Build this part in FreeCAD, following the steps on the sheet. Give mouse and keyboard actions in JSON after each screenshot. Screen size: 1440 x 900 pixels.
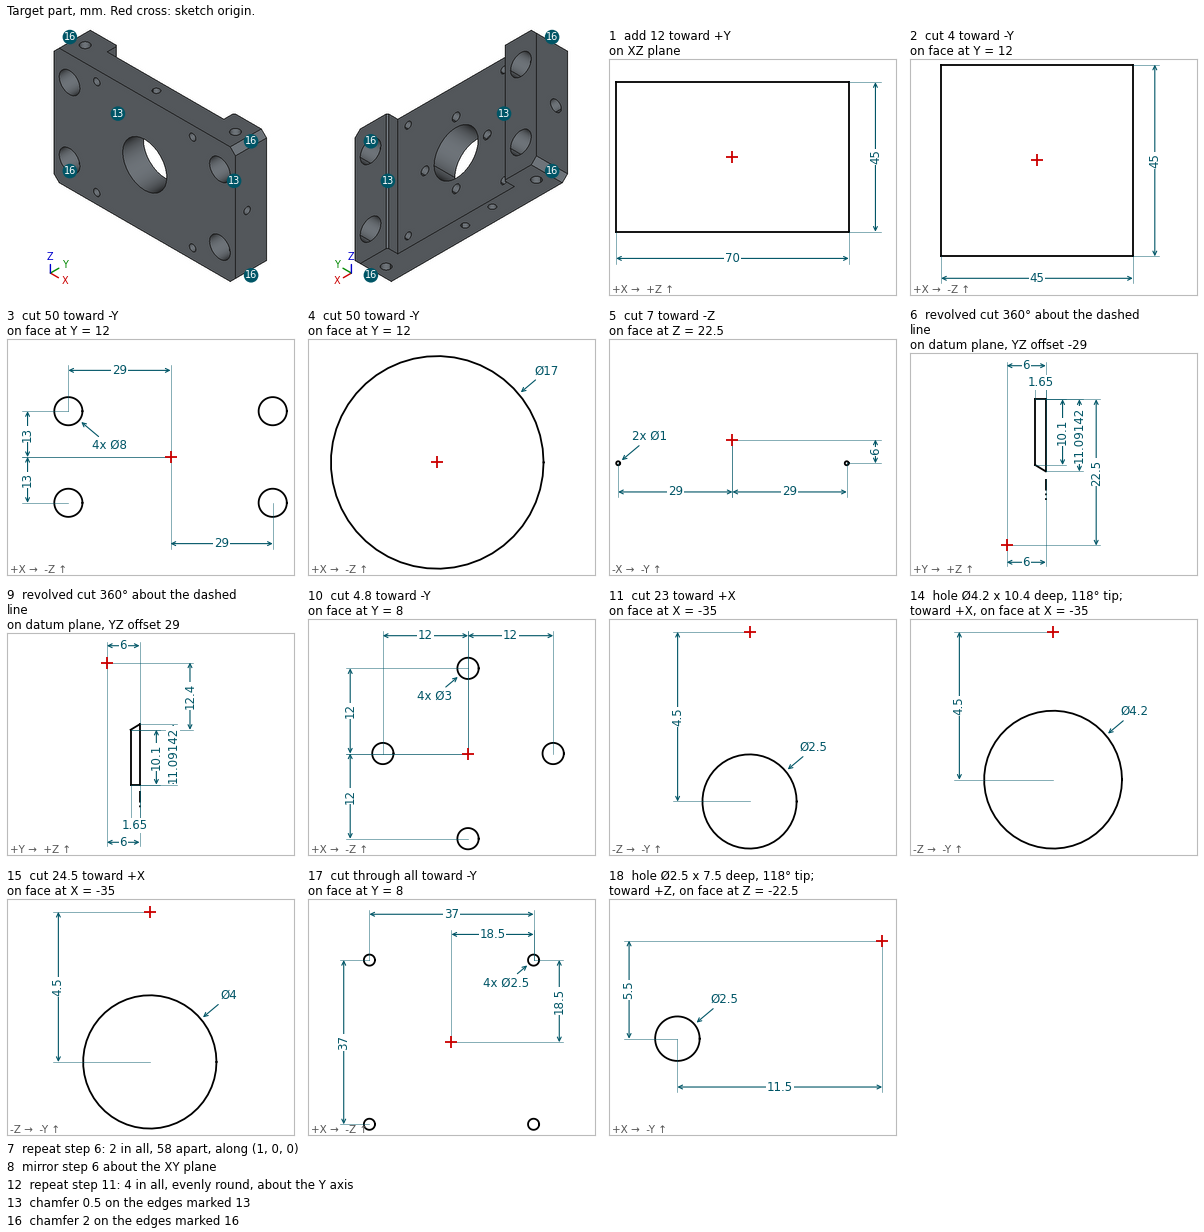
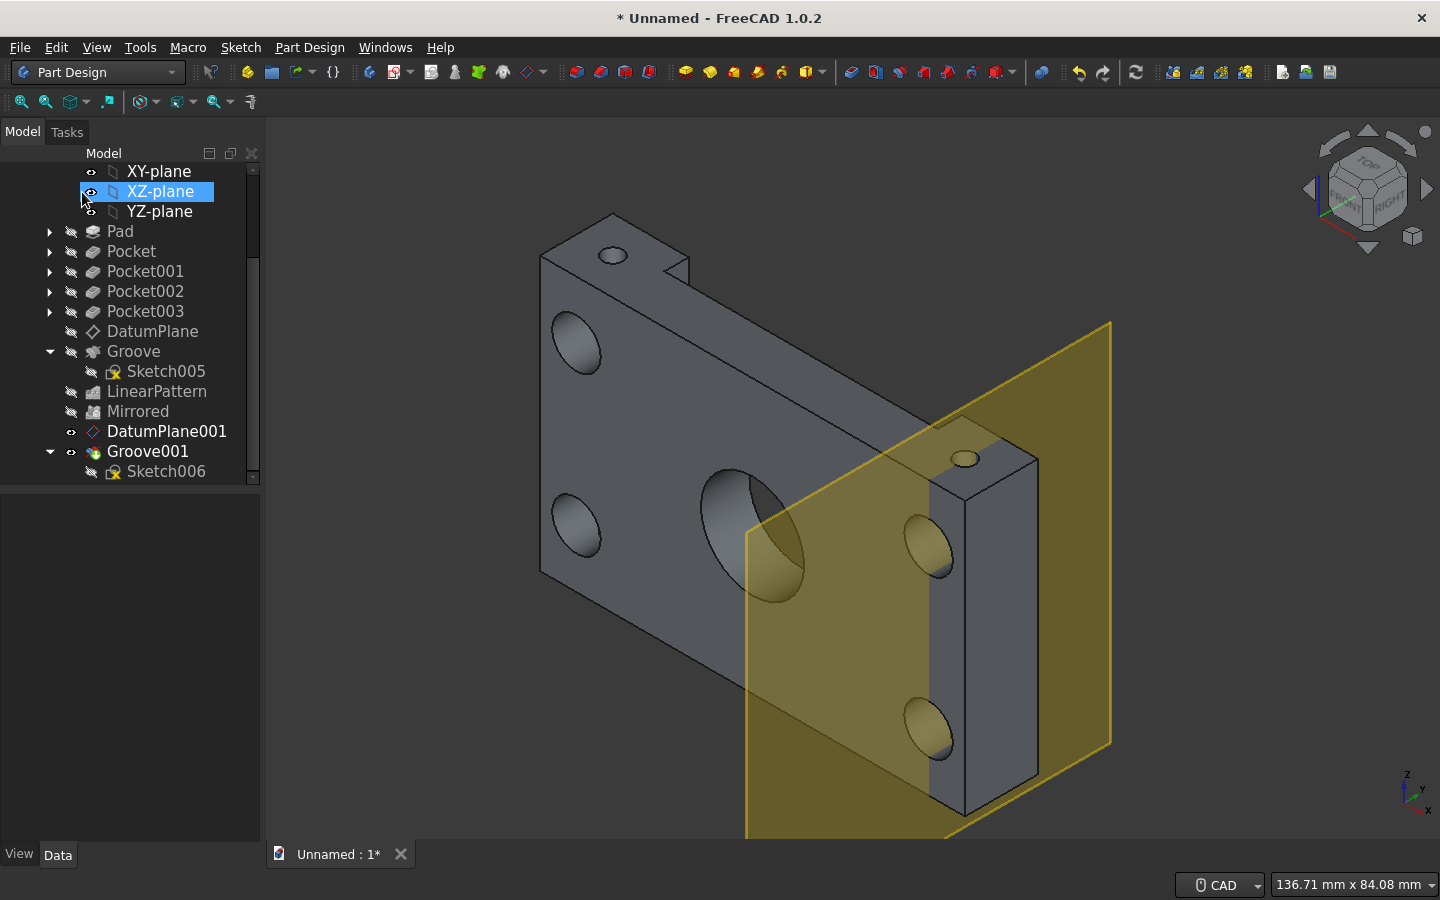
{"action": "left_click", "coordinate": [116, 432]}
{"action": "key", "text": "space"}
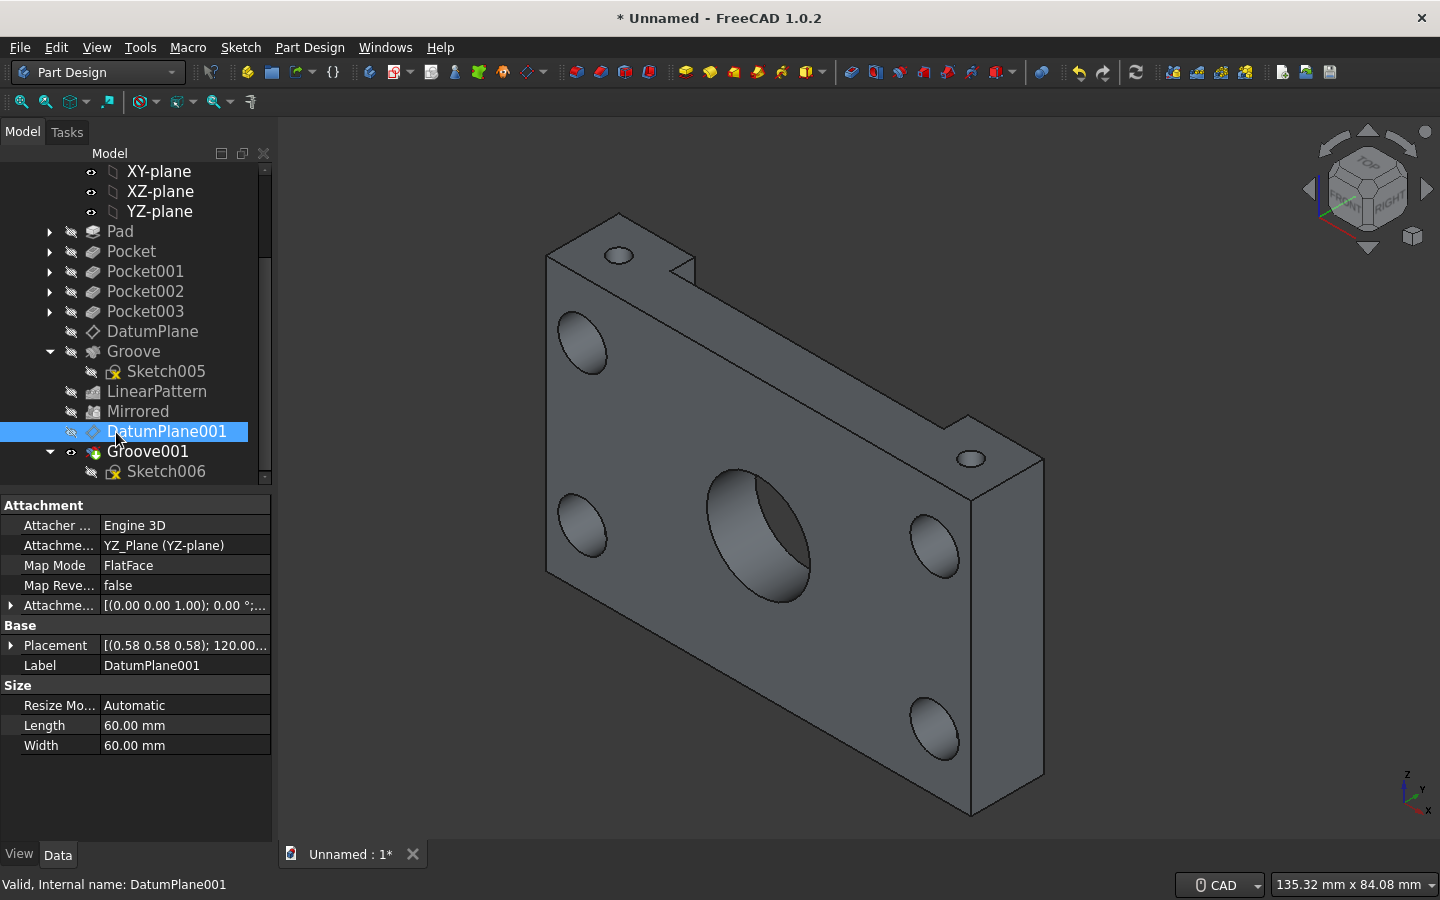
{"action": "key", "text": "4"}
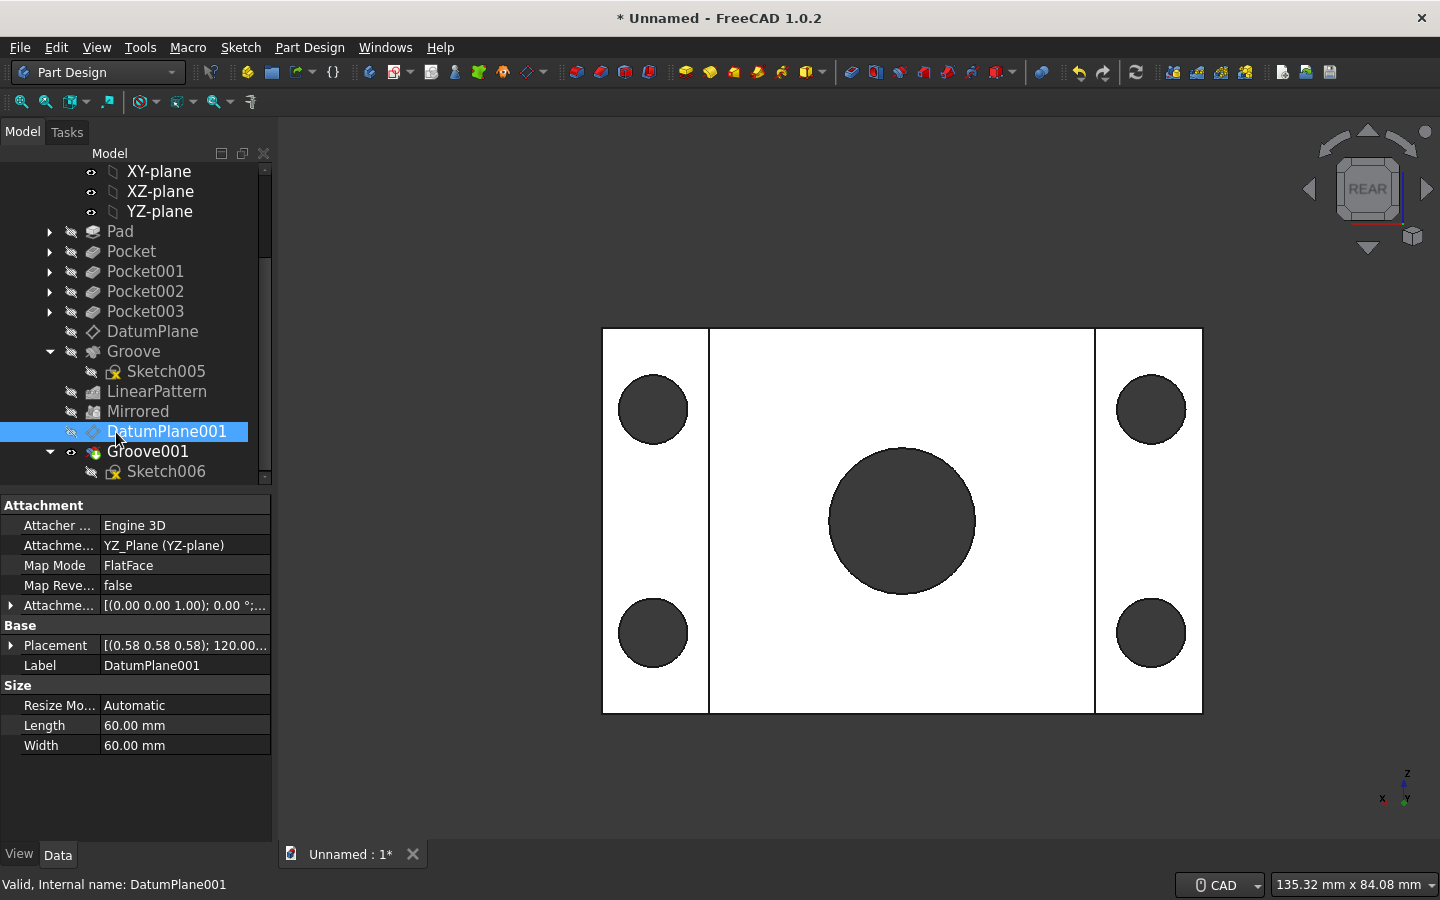
{"action": "left_click", "coordinate": [792, 410]}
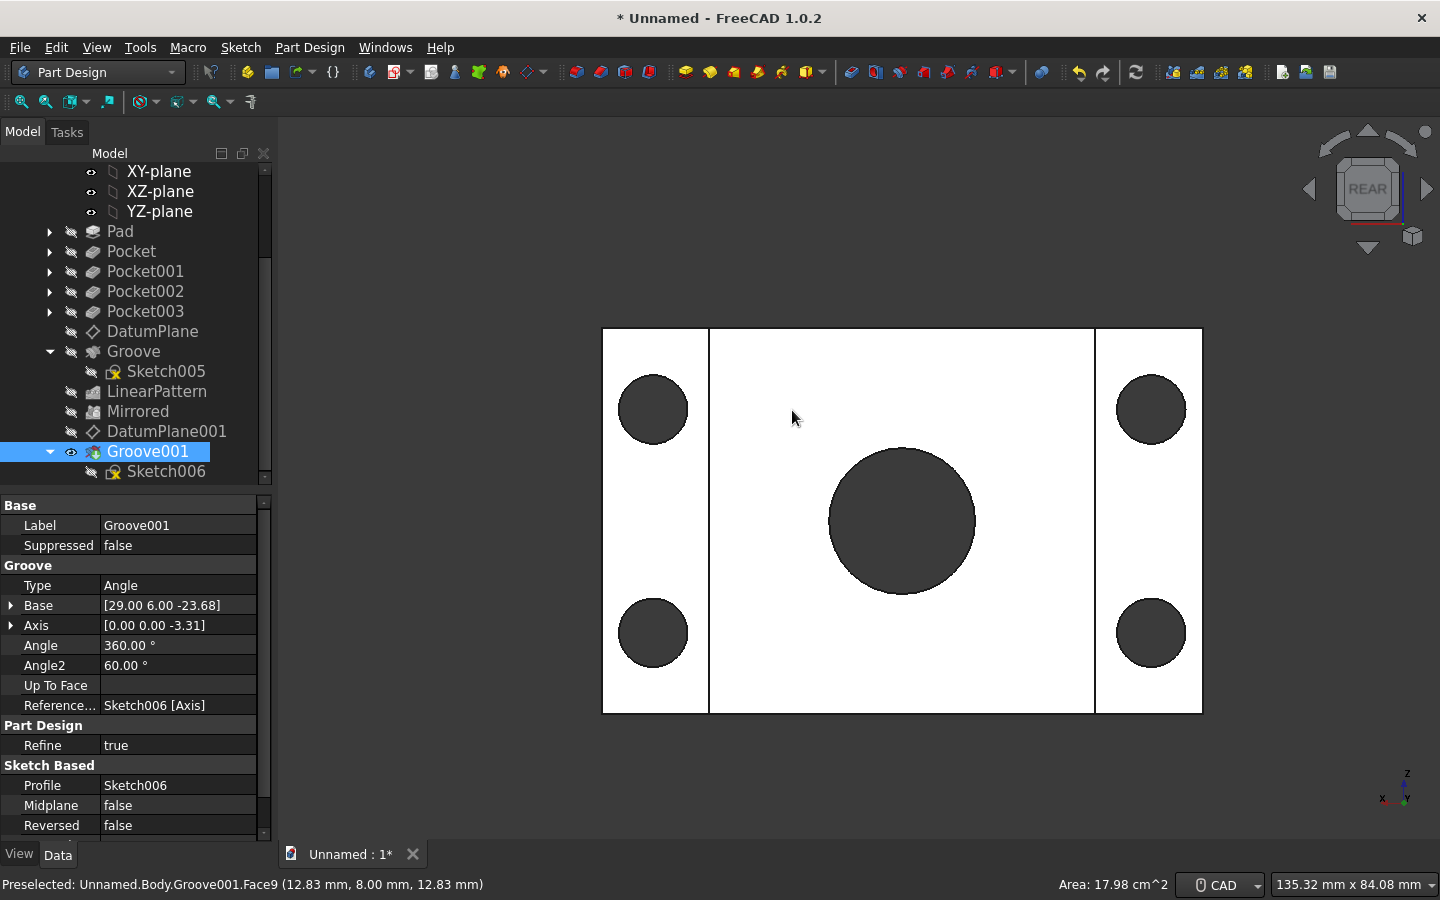
{"action": "left_click", "coordinate": [394, 72]}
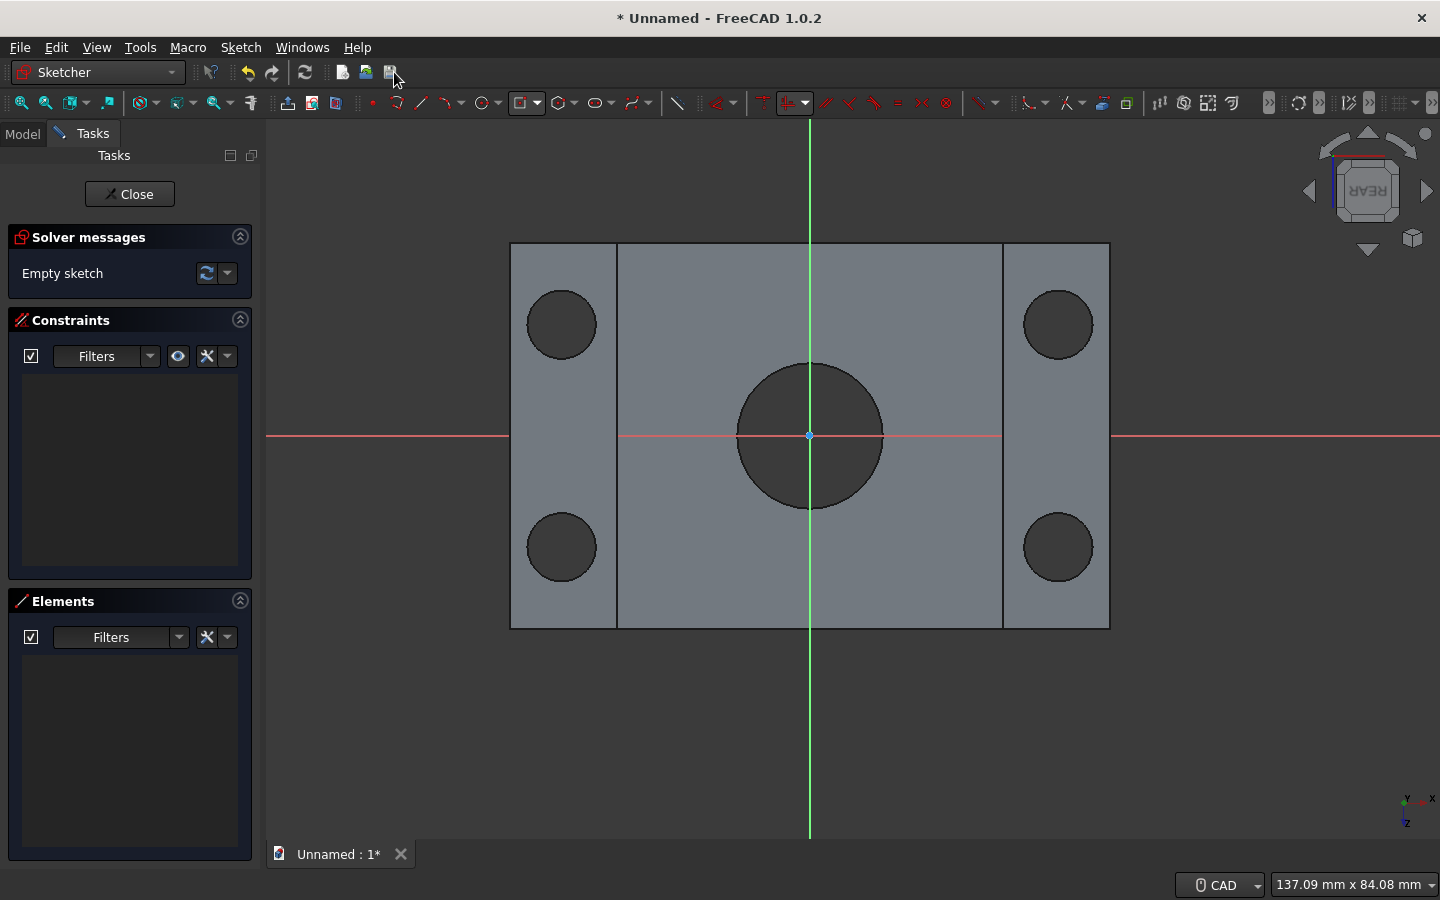
{"action": "left_click", "coordinate": [336, 104]}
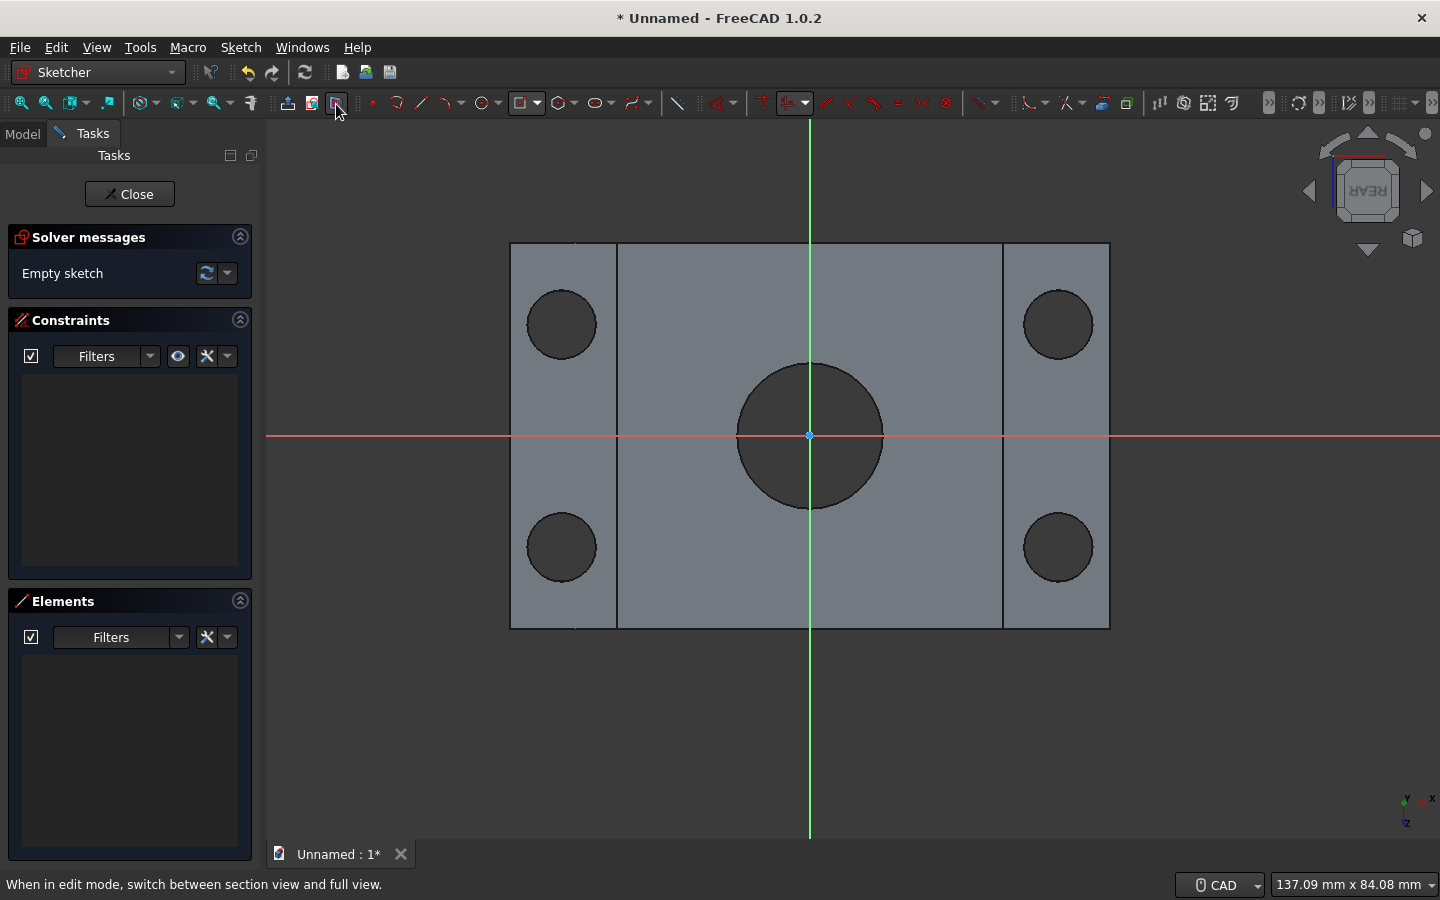
{"action": "scroll", "coordinate": [831, 401], "scroll_direction": "up", "scroll_amount": 4}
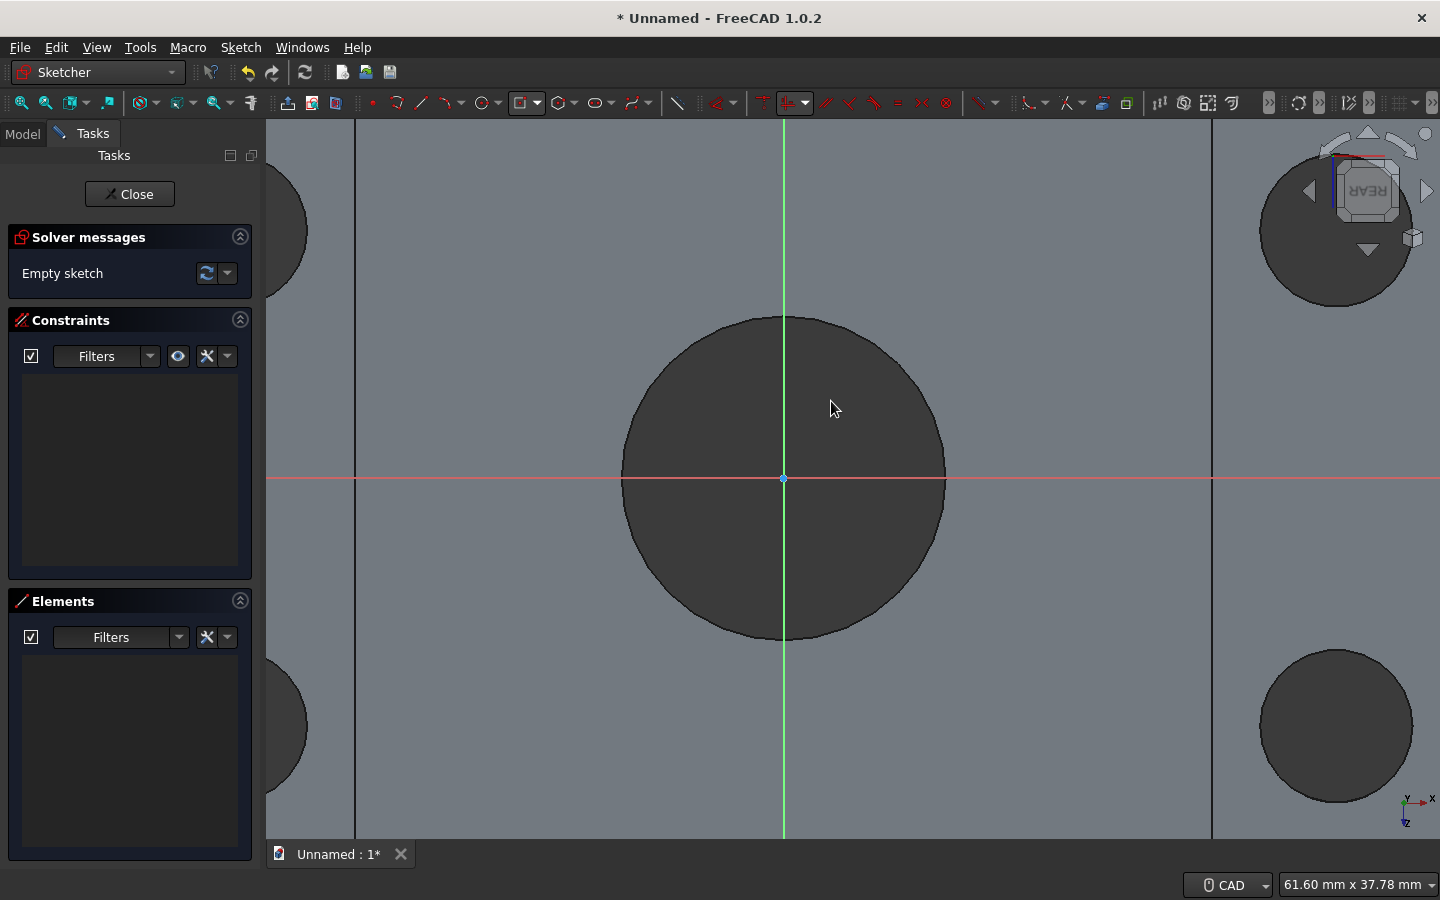
{"action": "left_click", "coordinate": [482, 104]}